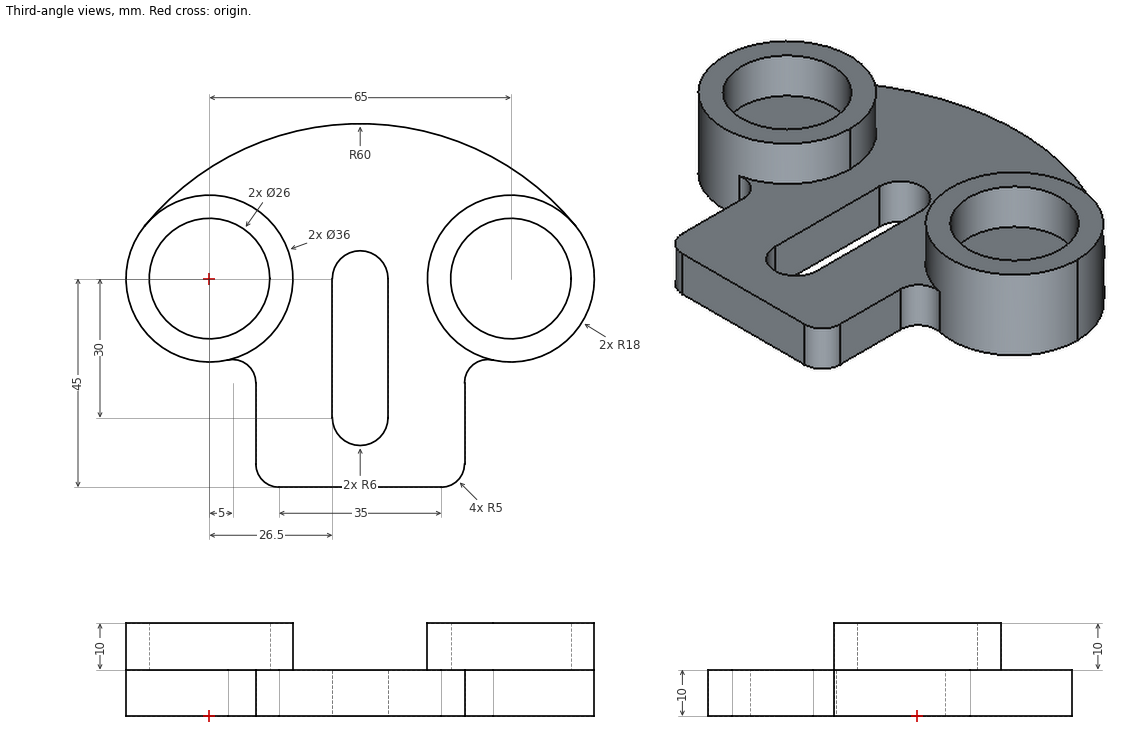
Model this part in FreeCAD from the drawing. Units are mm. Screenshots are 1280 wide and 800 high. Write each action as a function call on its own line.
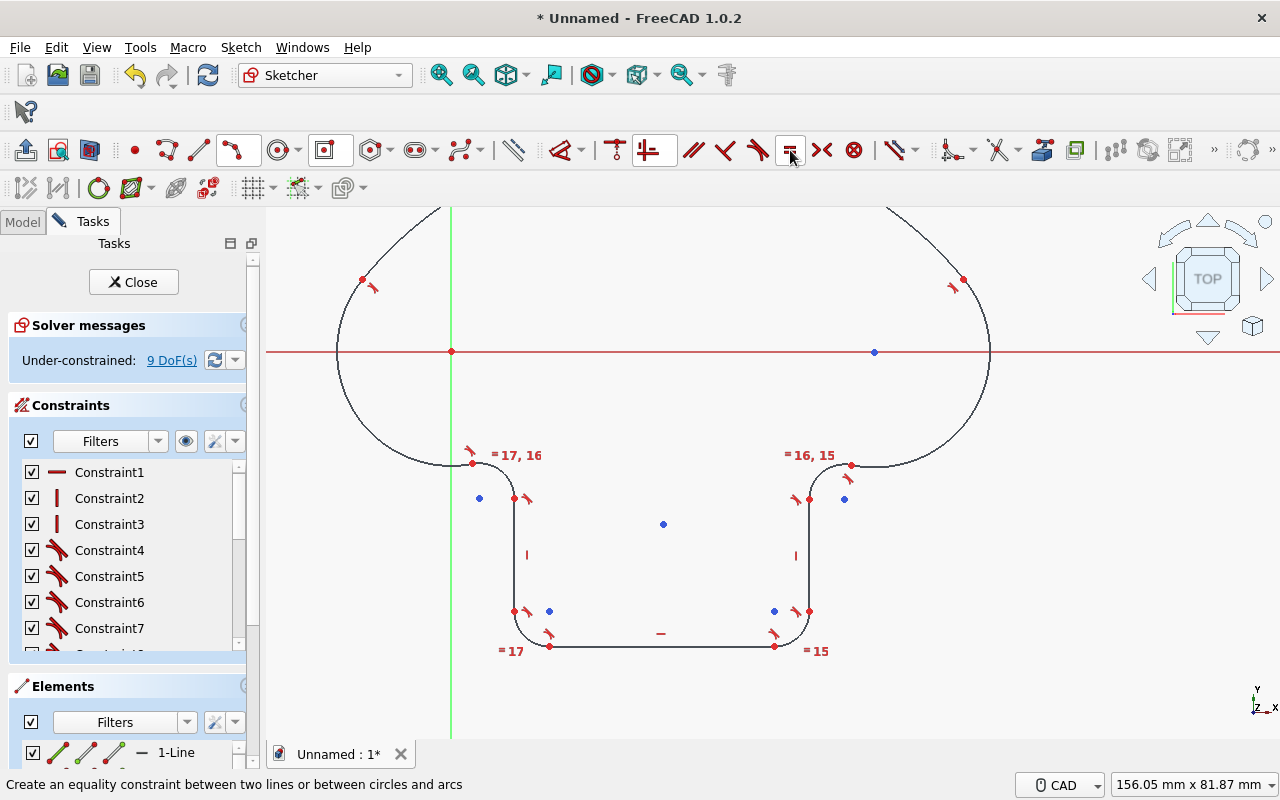
click(934, 451)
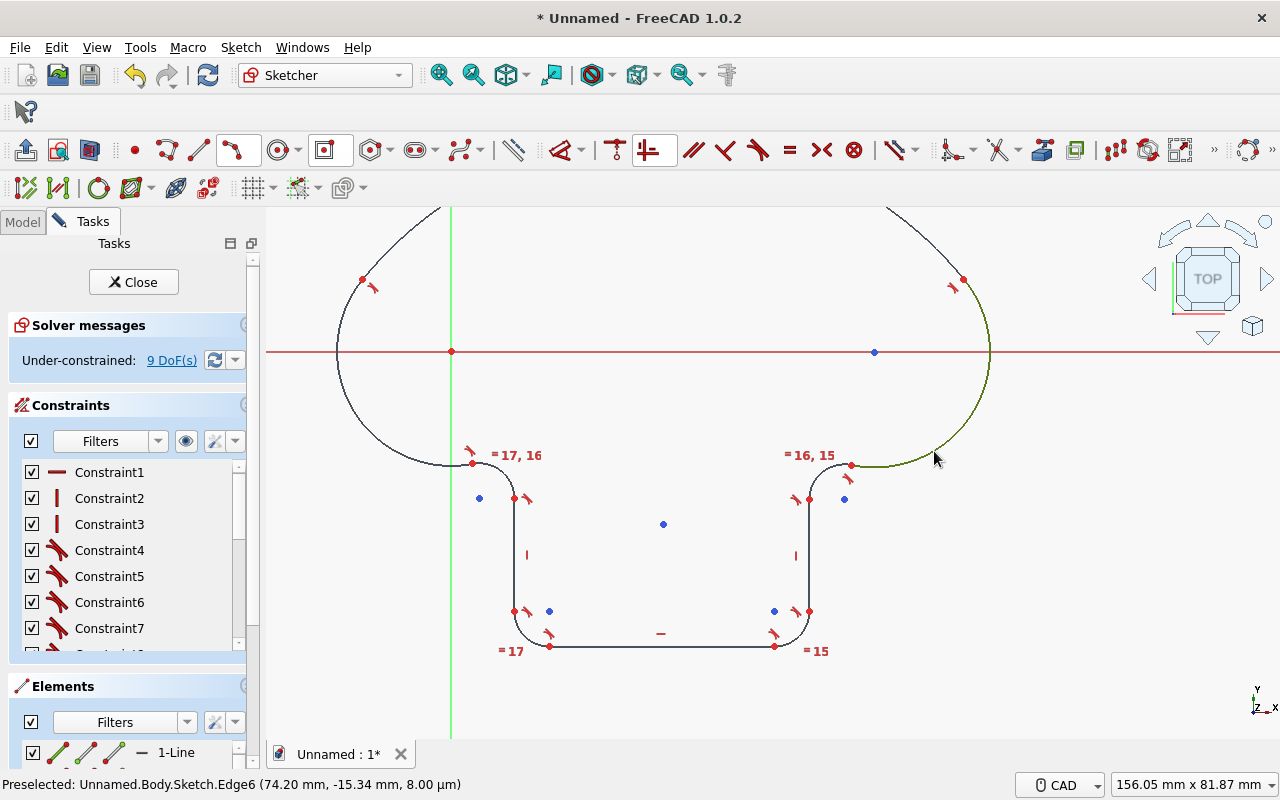
click(392, 449)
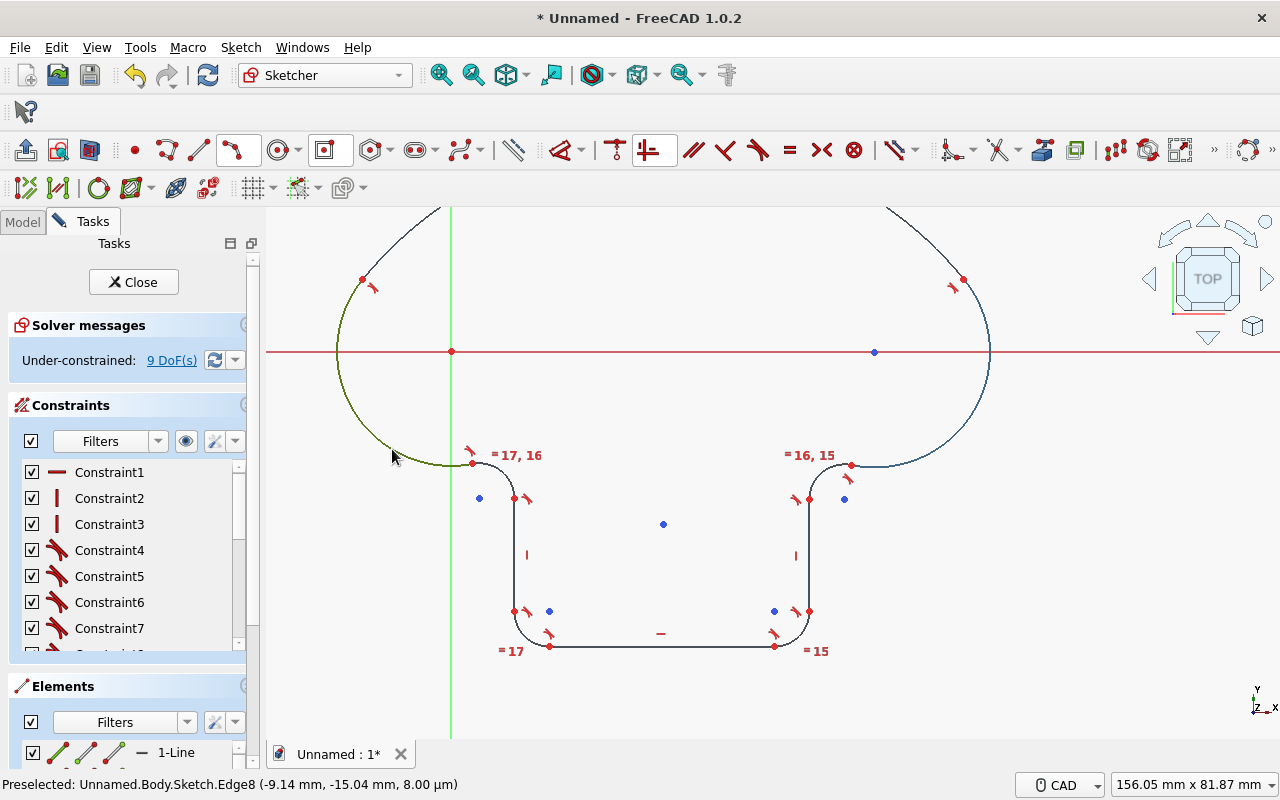
click(790, 150)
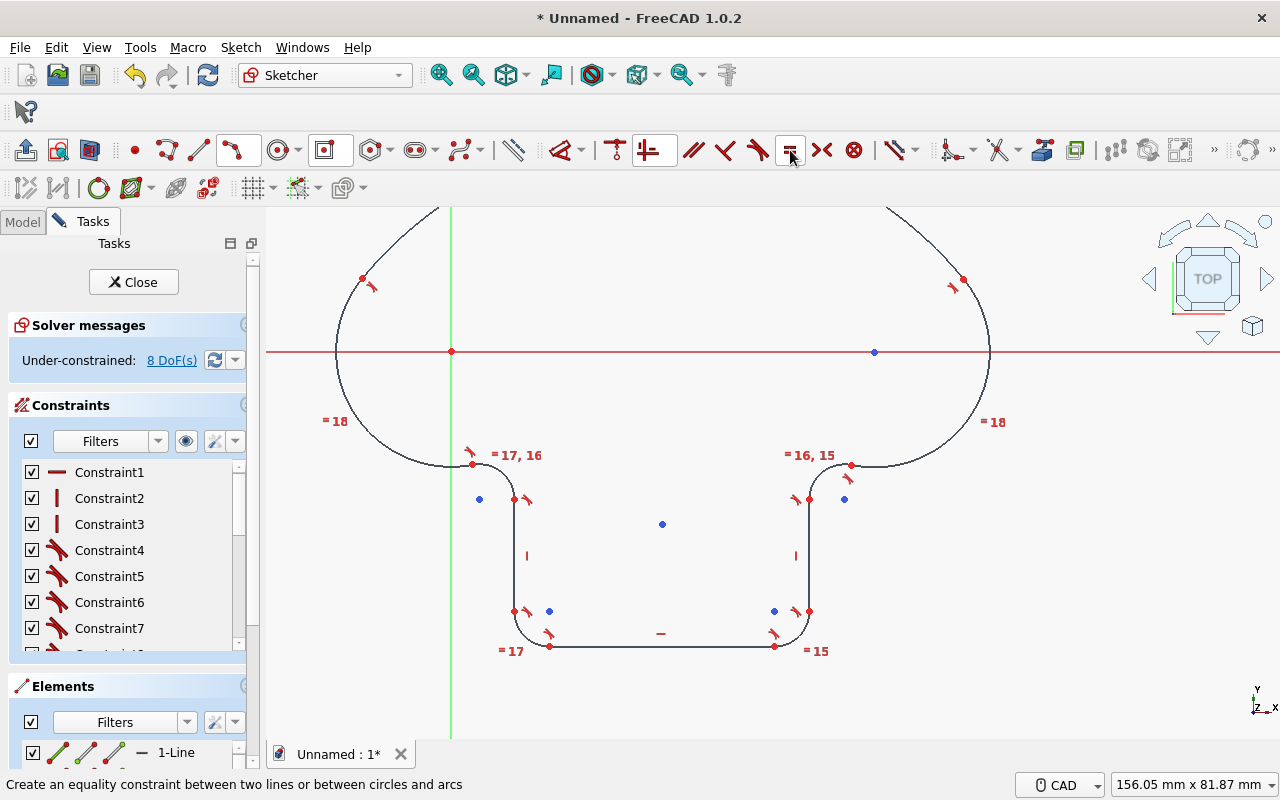
click(875, 352)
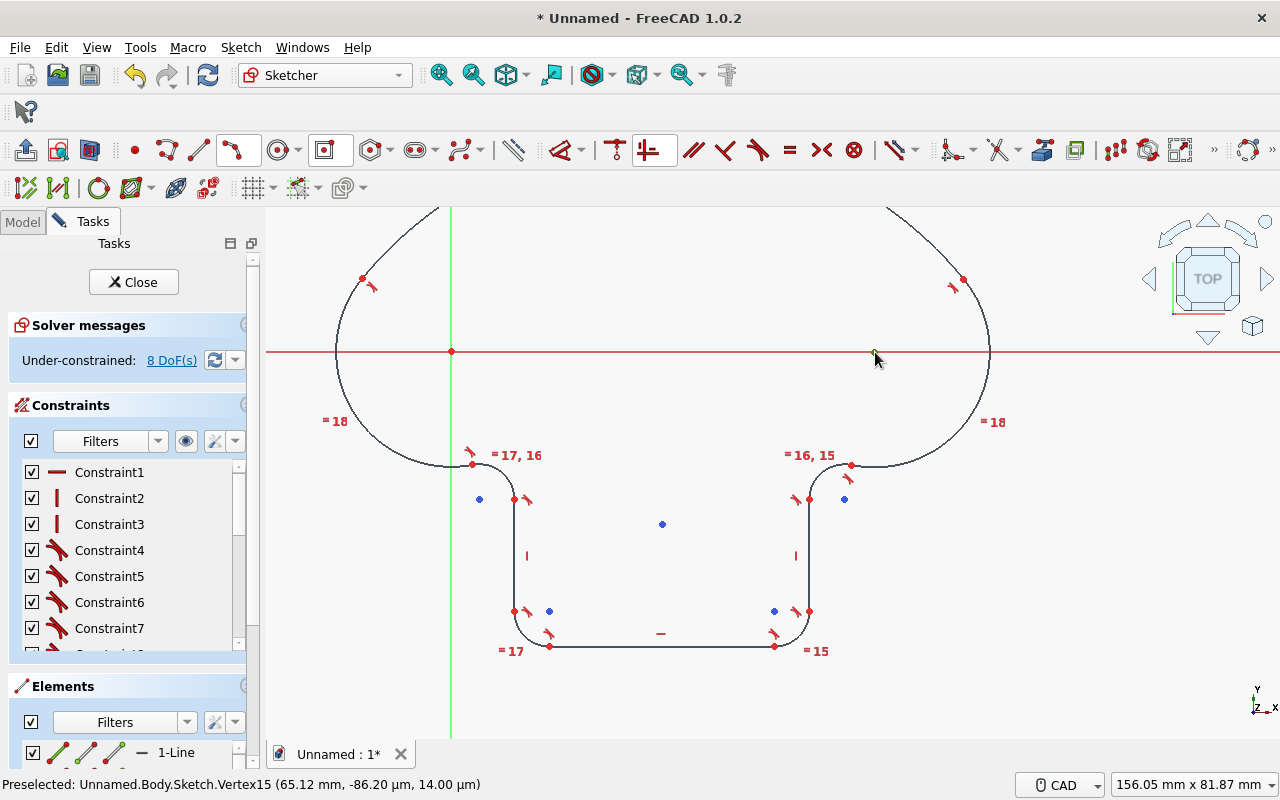
click(411, 352)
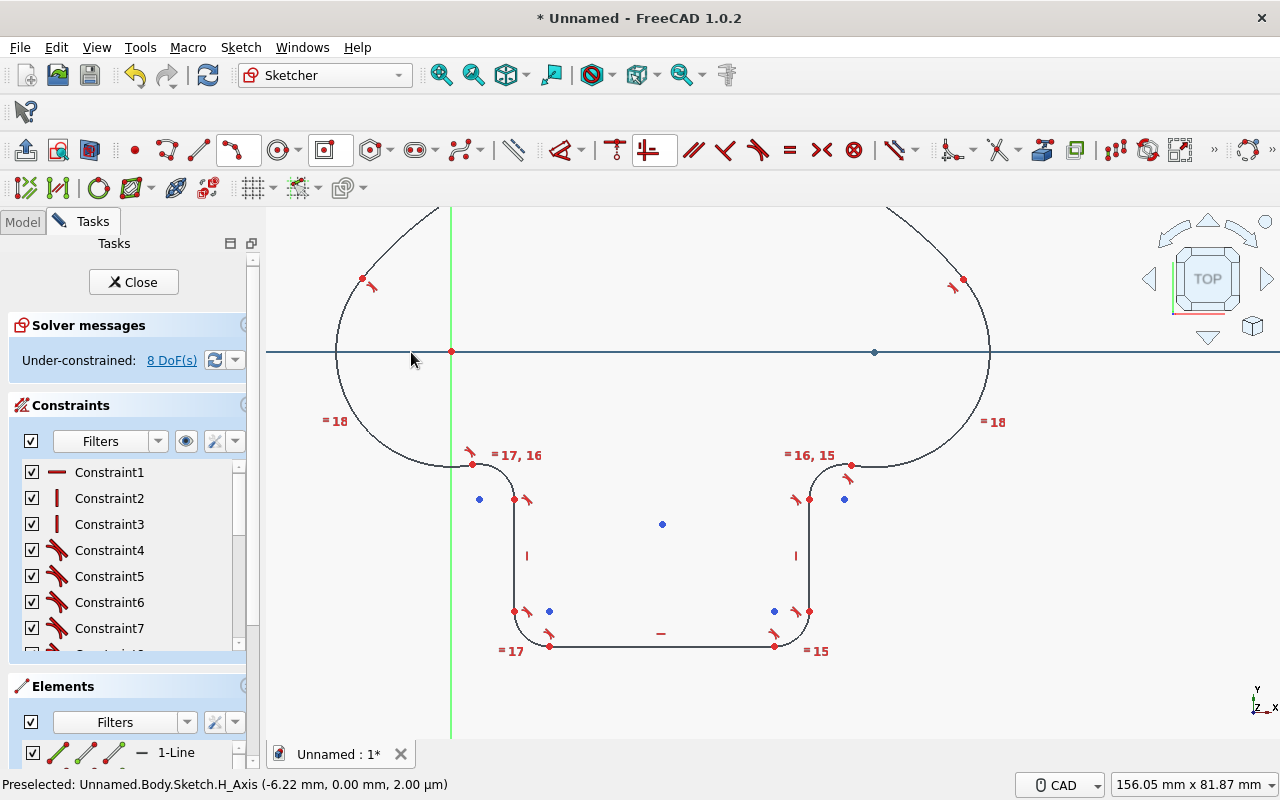
click(616, 150)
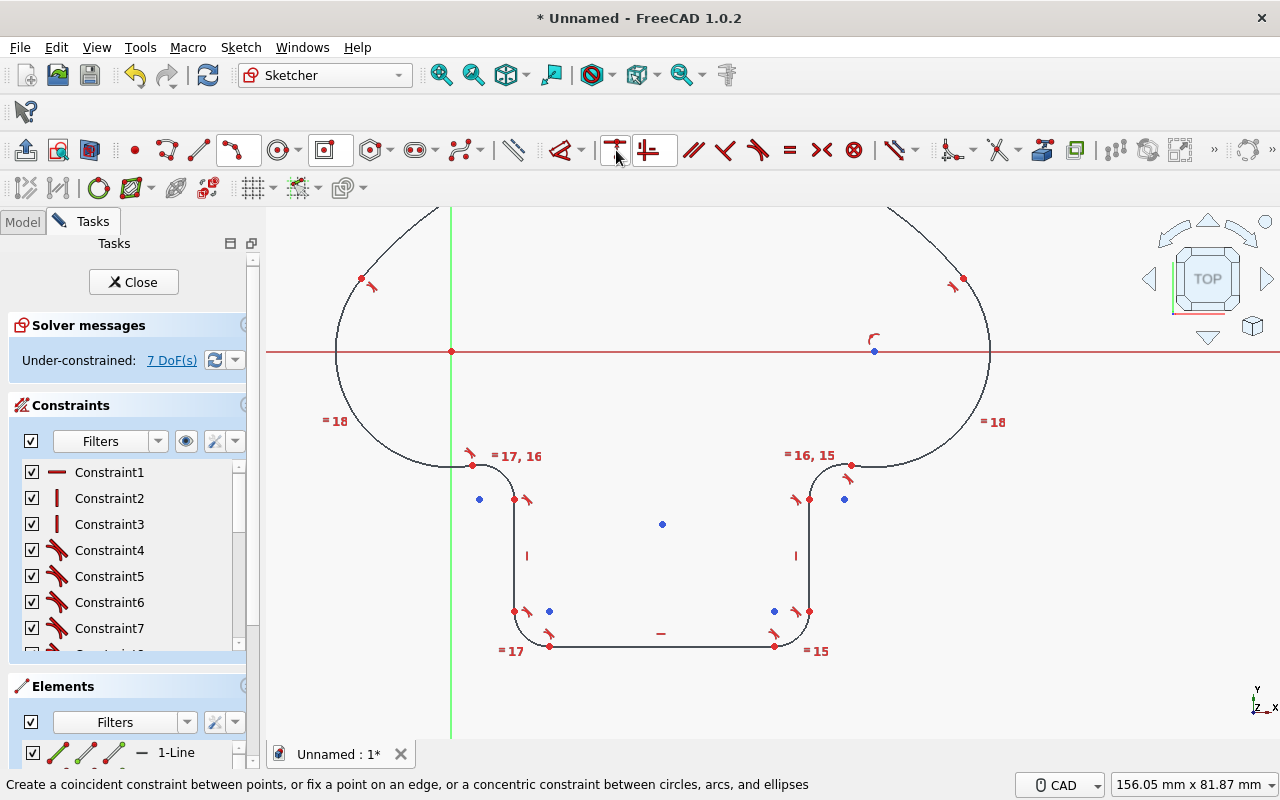
scroll(790, 643, up, 2)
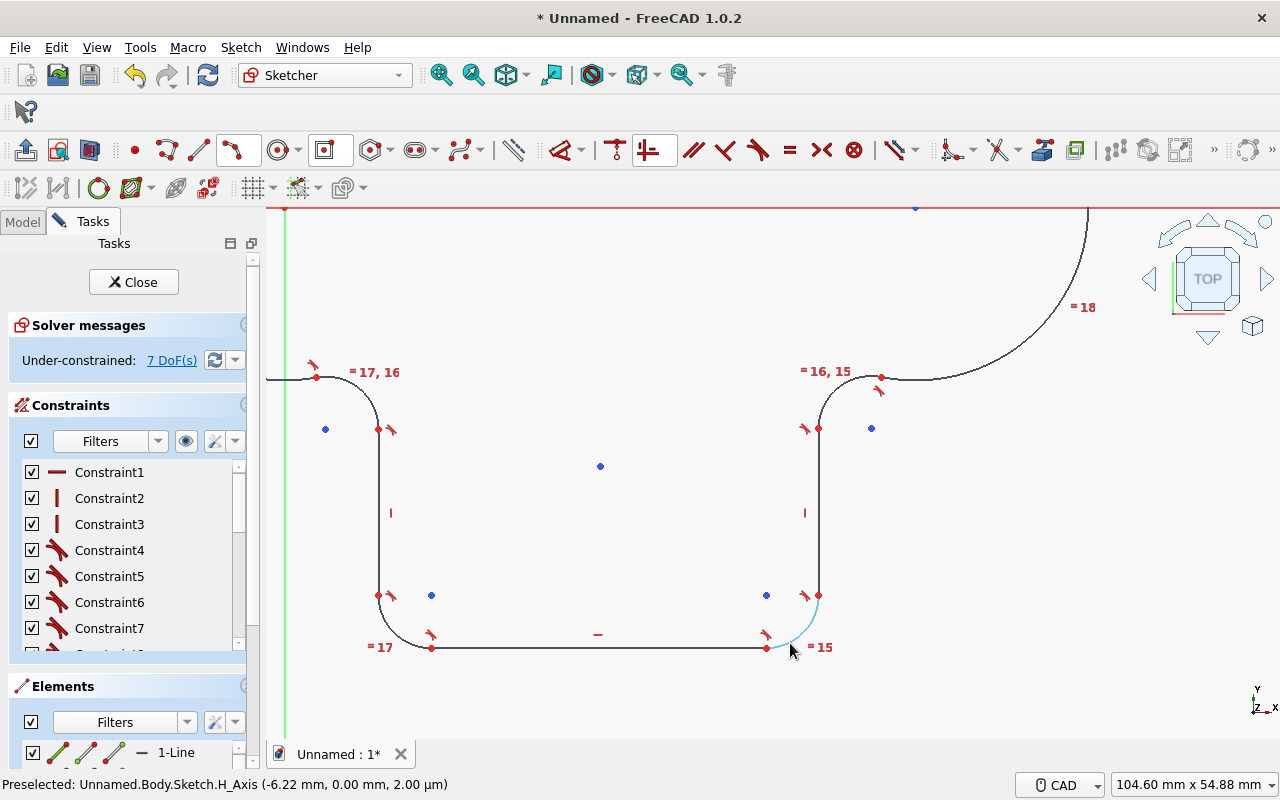
click(790, 642)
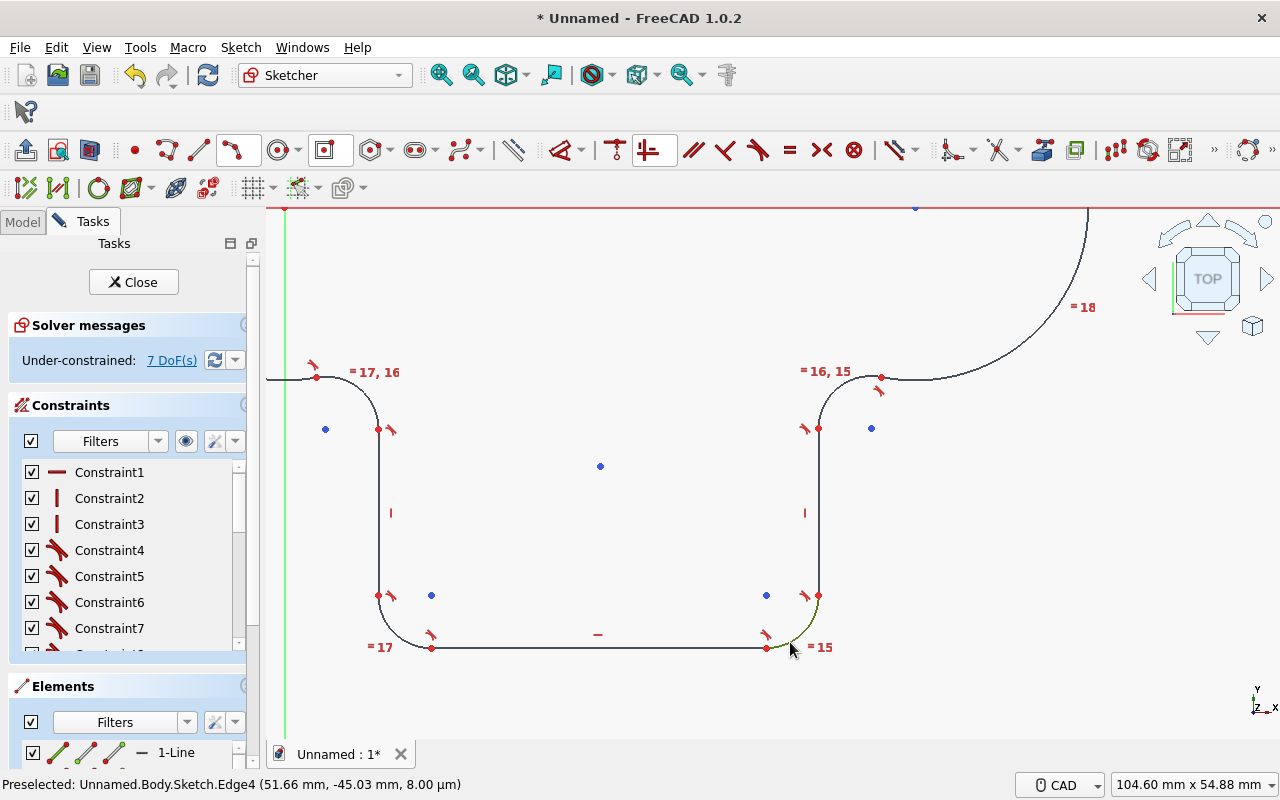
click(584, 150)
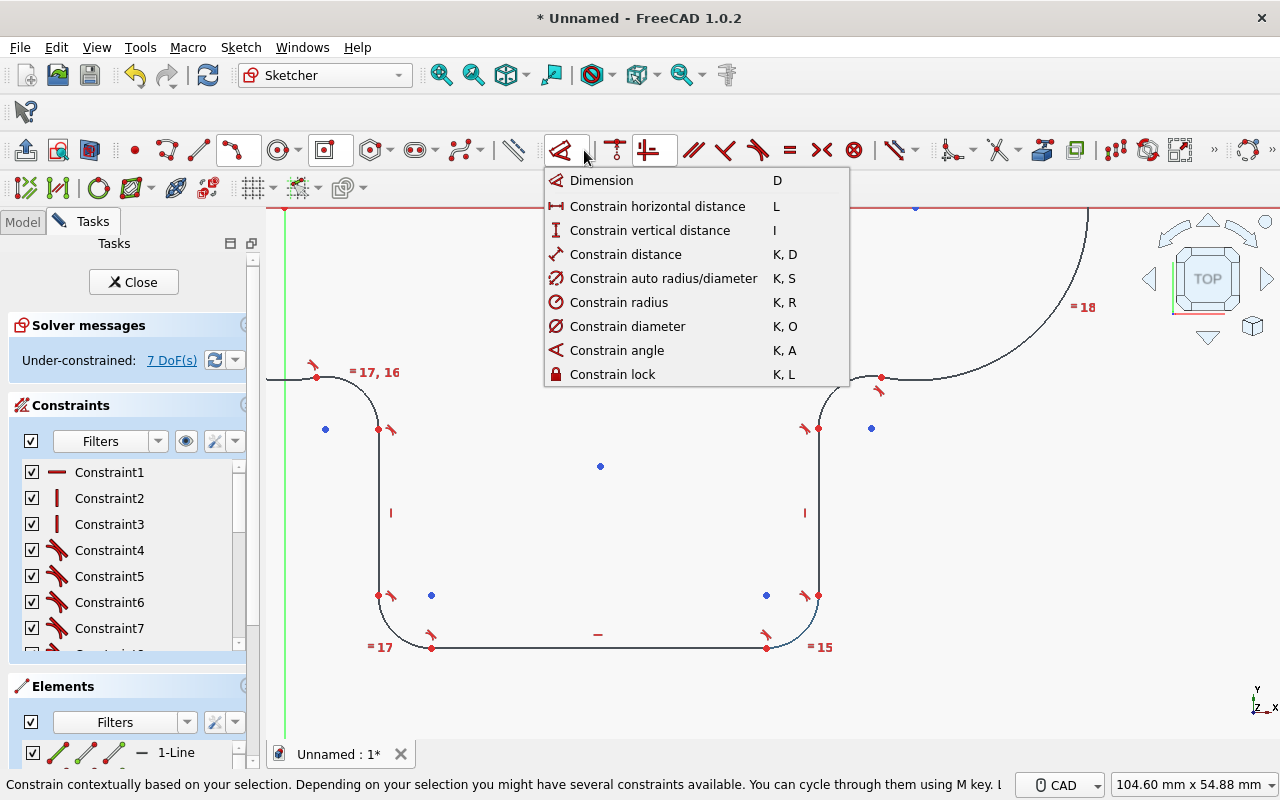
click(697, 302)